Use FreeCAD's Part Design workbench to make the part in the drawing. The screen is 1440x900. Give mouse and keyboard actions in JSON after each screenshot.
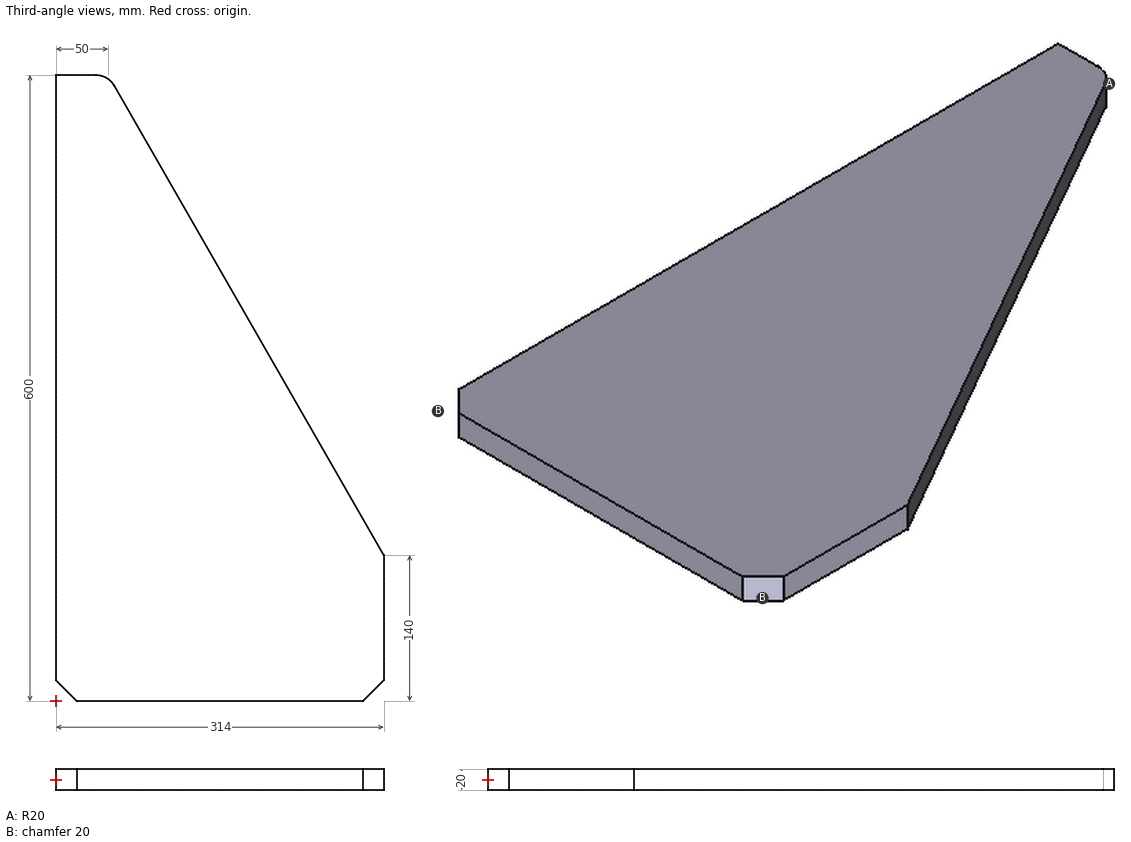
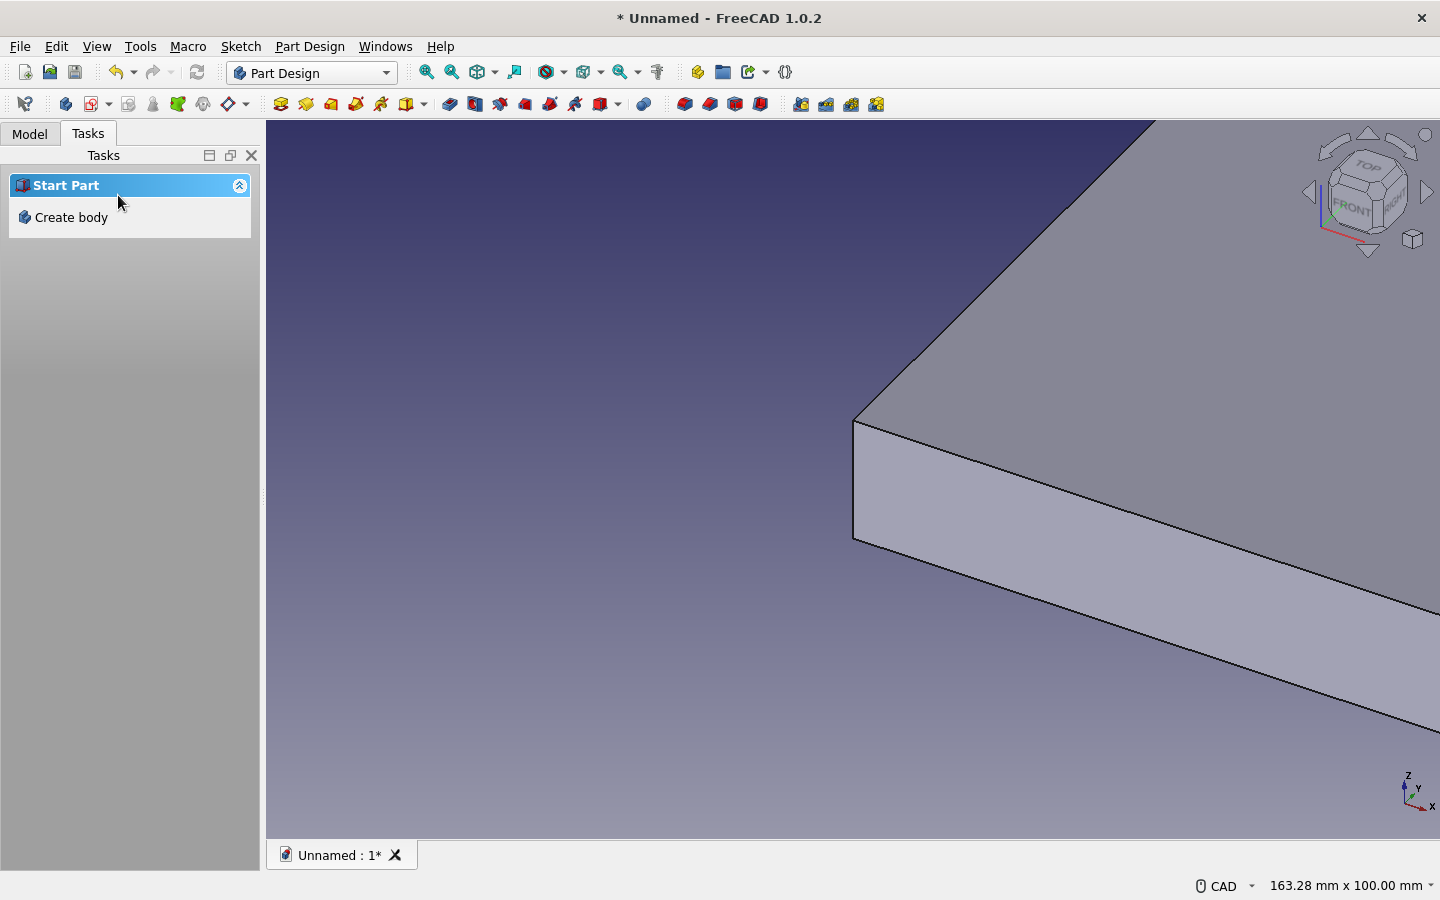
{"action": "key", "text": "v f"}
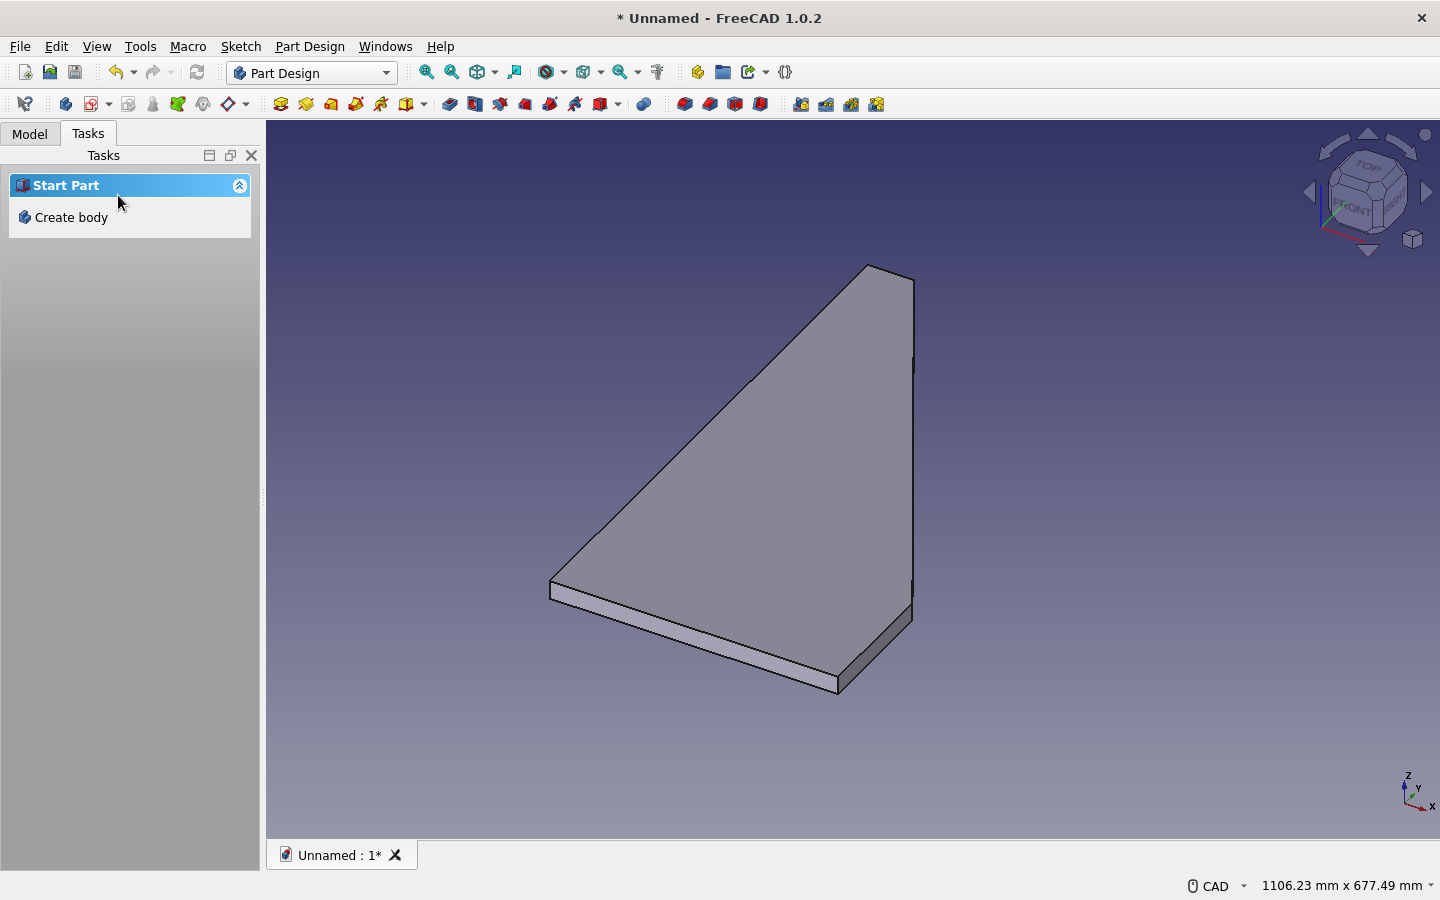
{"action": "scroll", "coordinate": [914, 288], "scroll_direction": "up", "scroll_amount": 4}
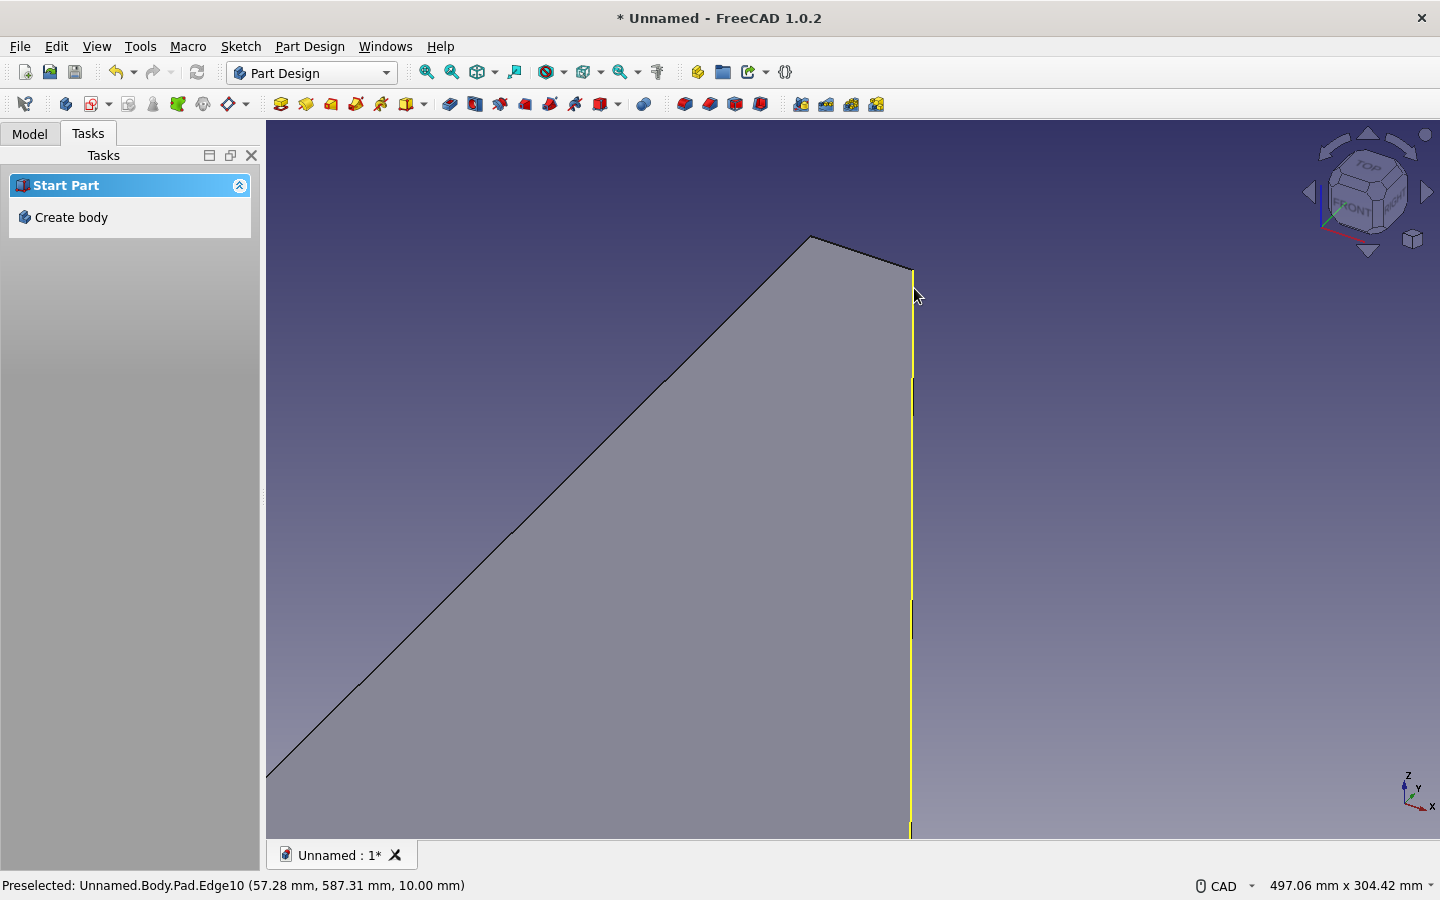
{"action": "left_click", "coordinate": [427, 72]}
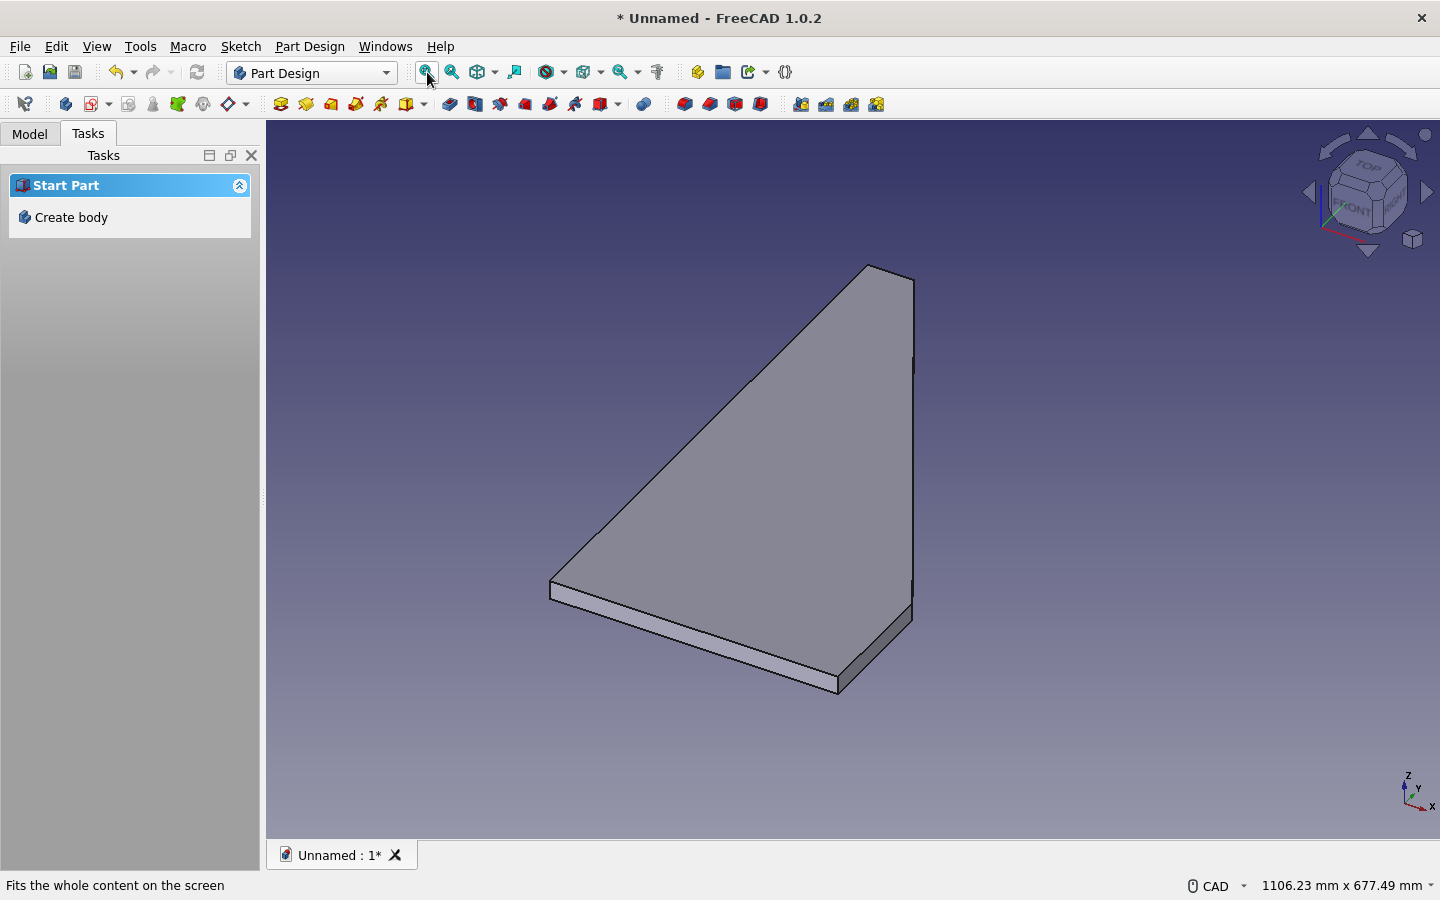
{"action": "key", "text": "0"}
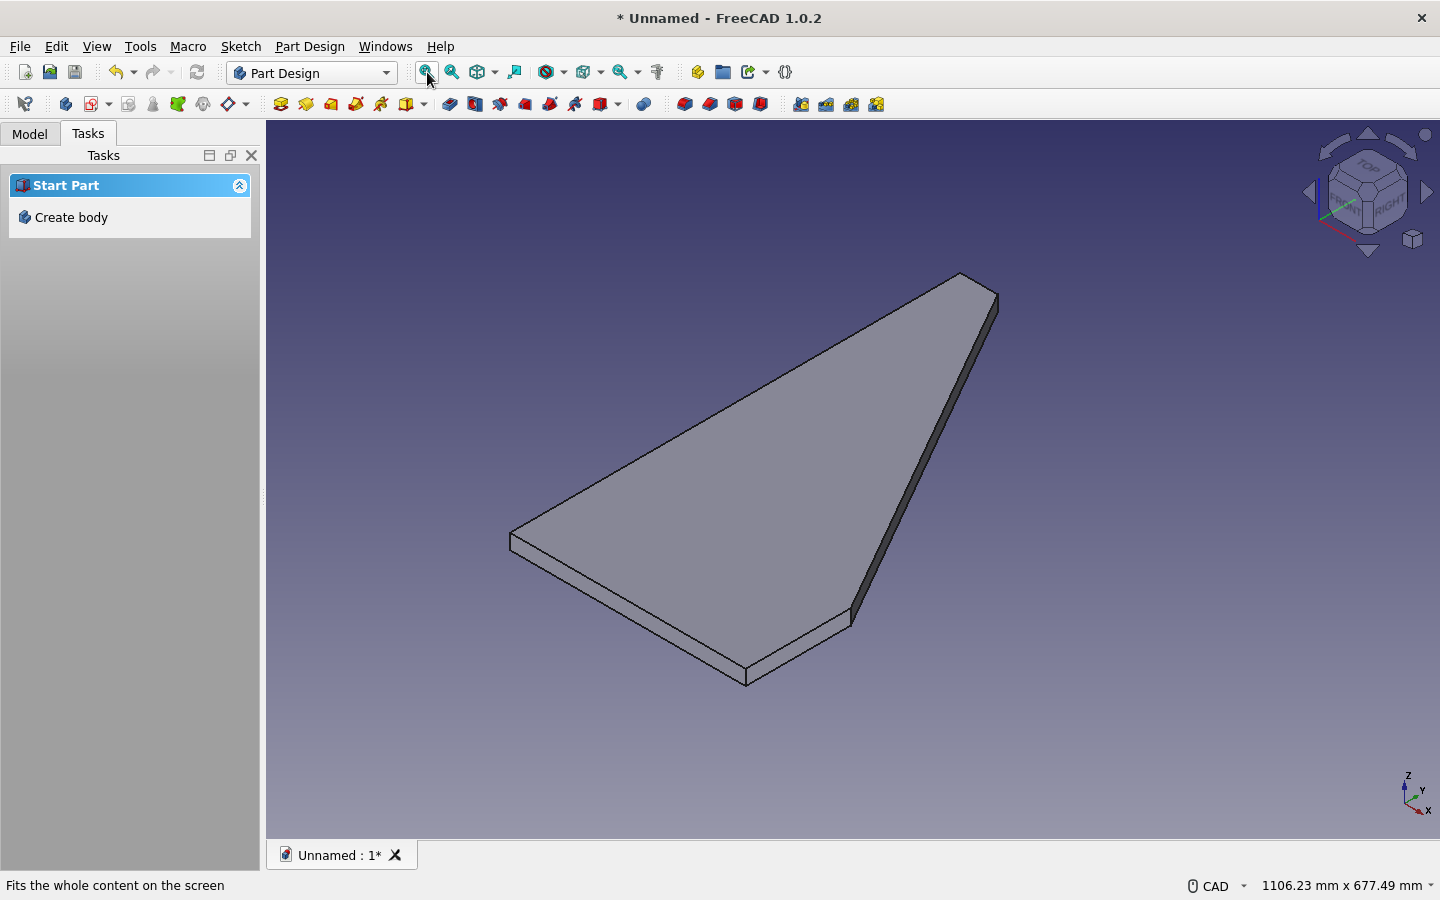
{"action": "scroll", "coordinate": [998, 302], "scroll_direction": "up", "scroll_amount": 4}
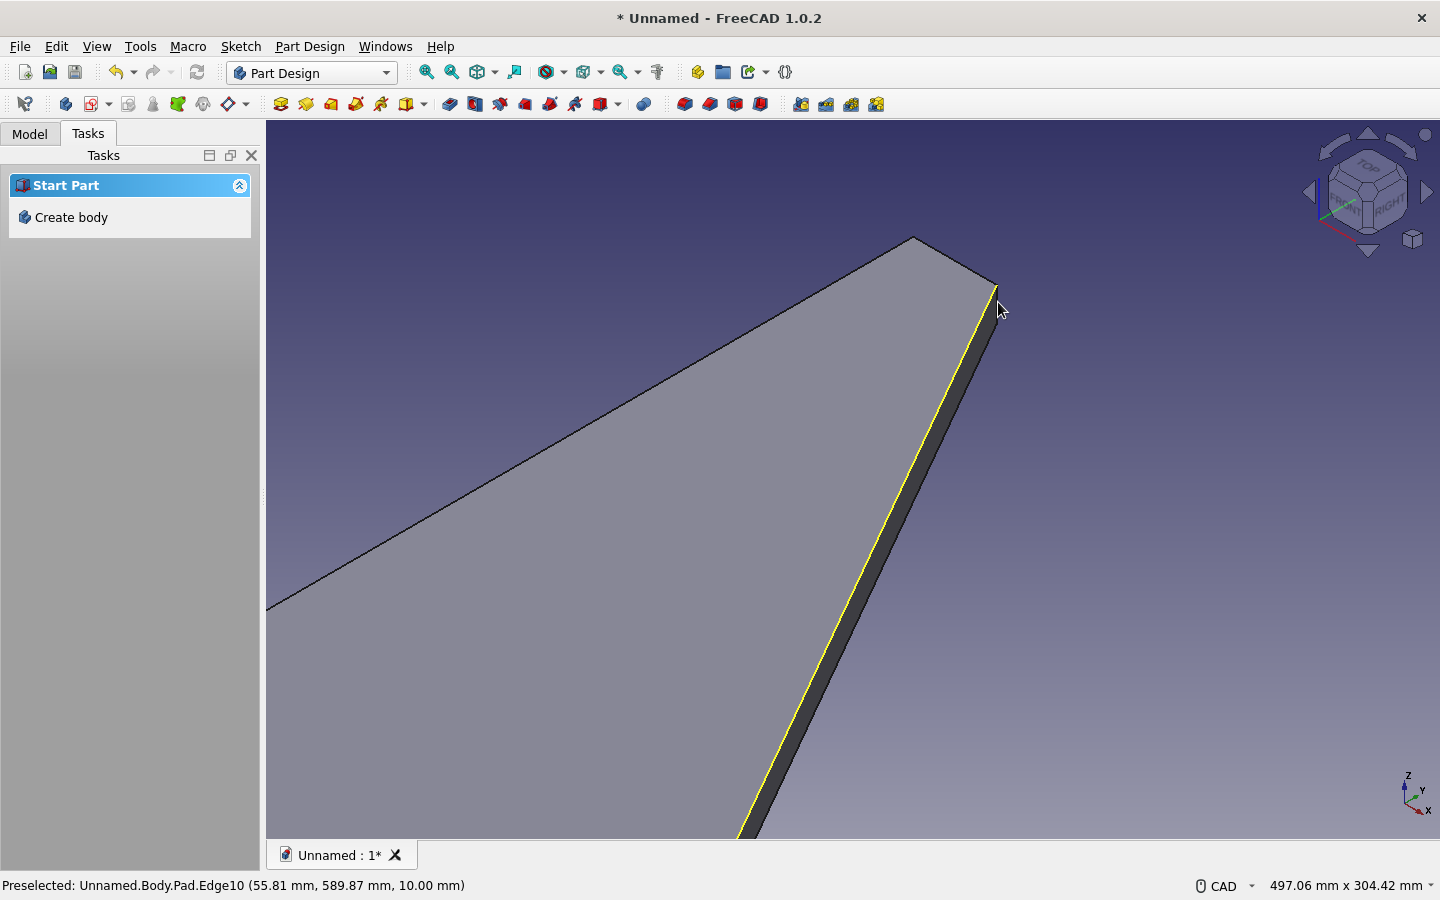
{"action": "key", "text": "v f"}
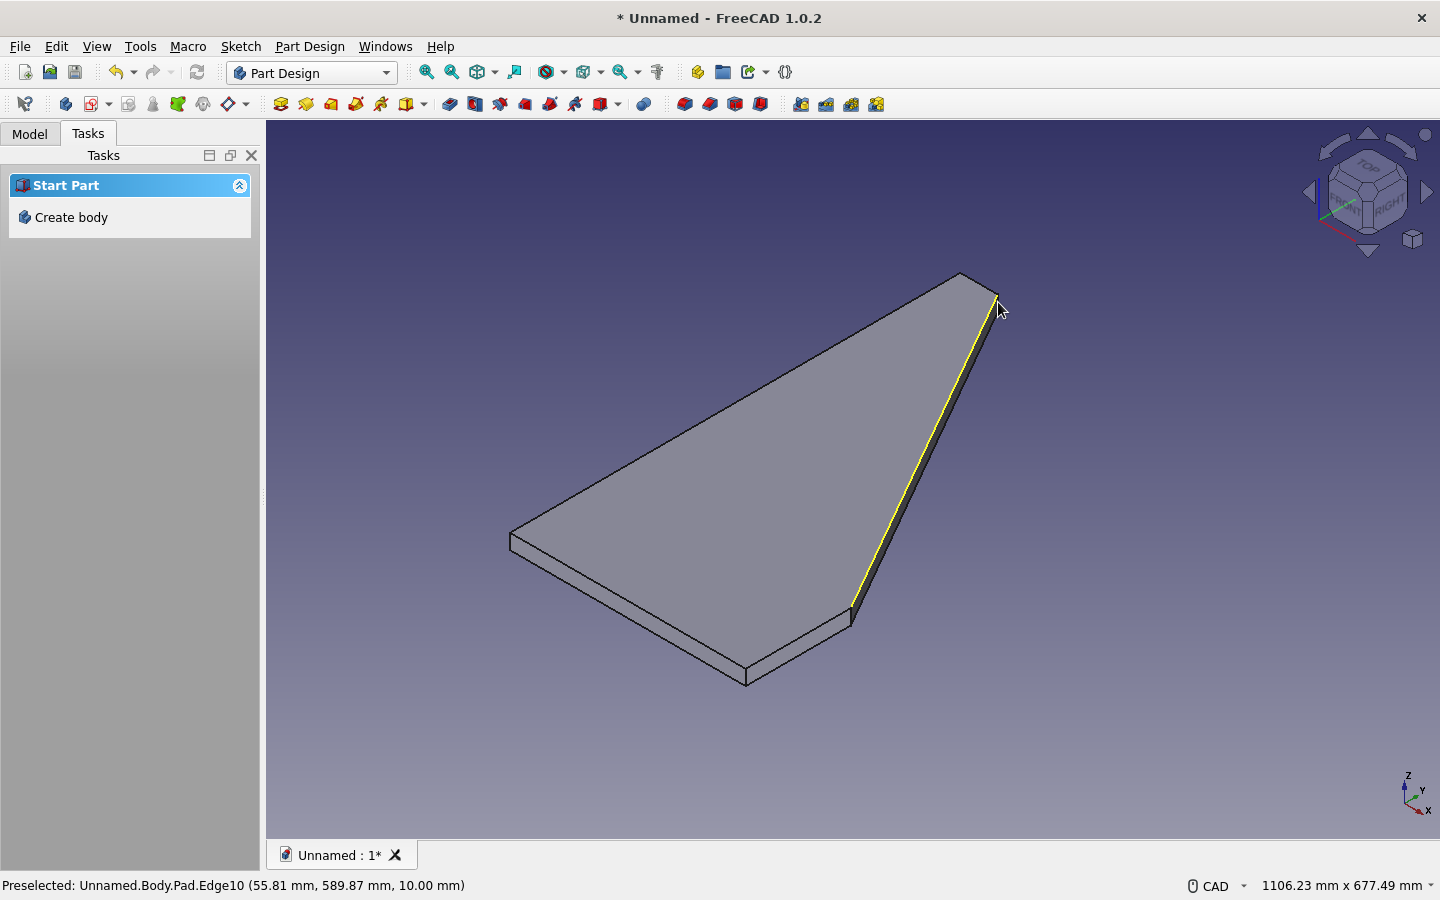
{"action": "key", "text": "2"}